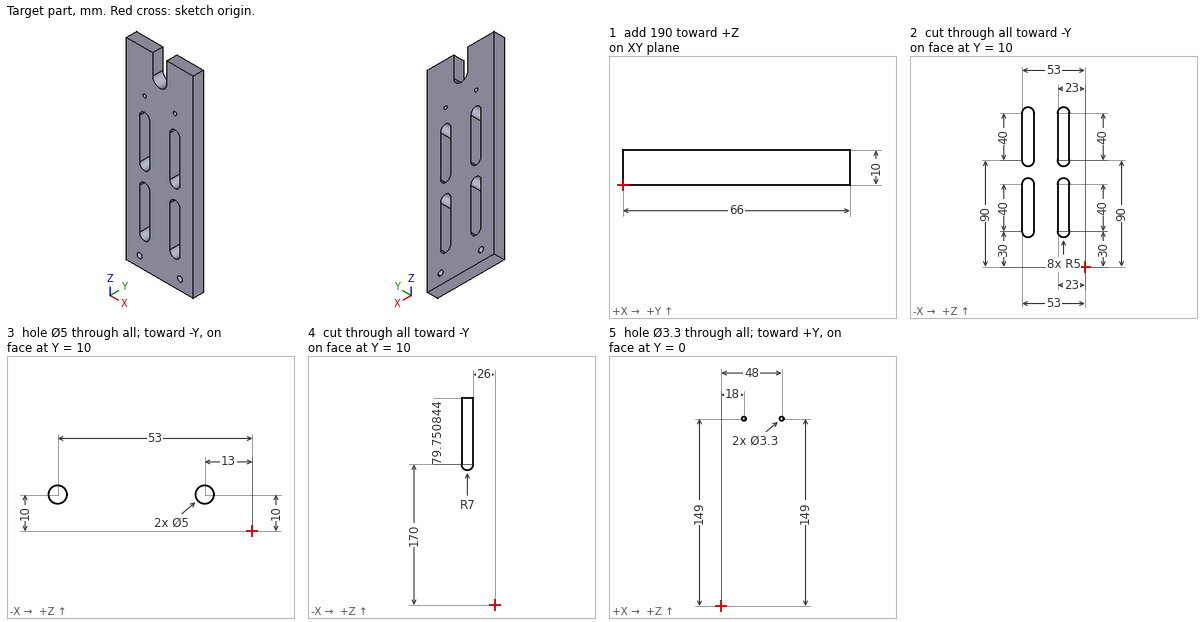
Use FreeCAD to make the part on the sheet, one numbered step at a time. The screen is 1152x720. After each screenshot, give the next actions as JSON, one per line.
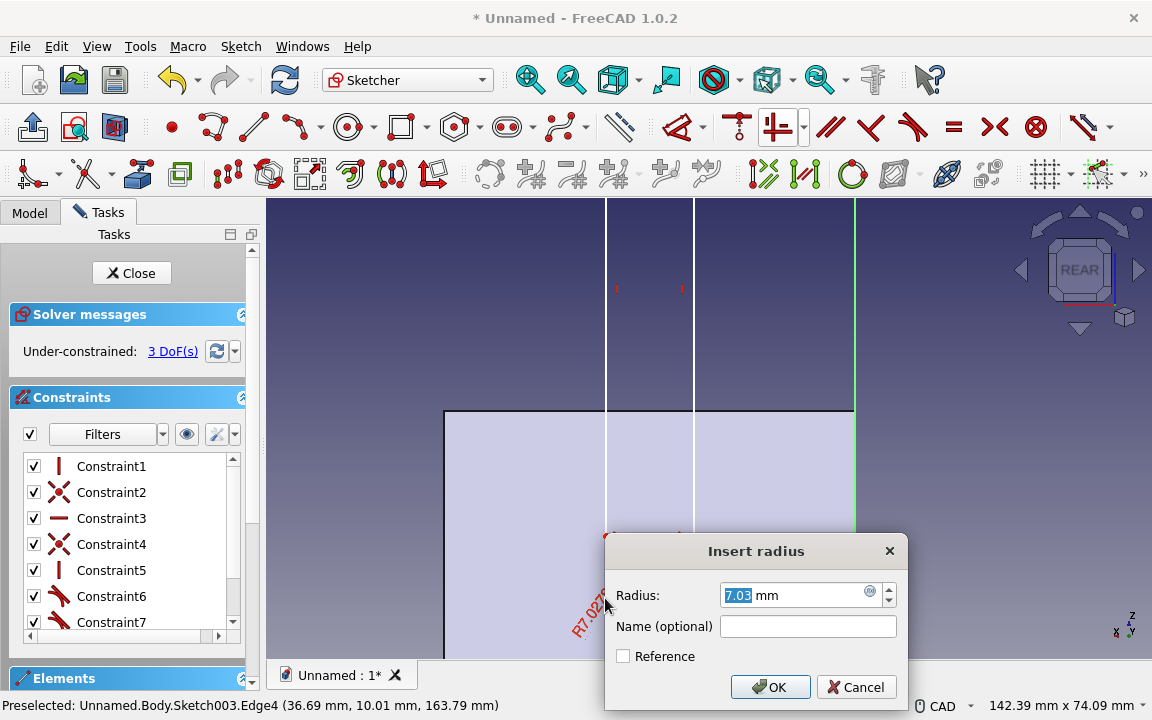
{"action": "type", "text": "7"}
{"action": "key", "text": "Return"}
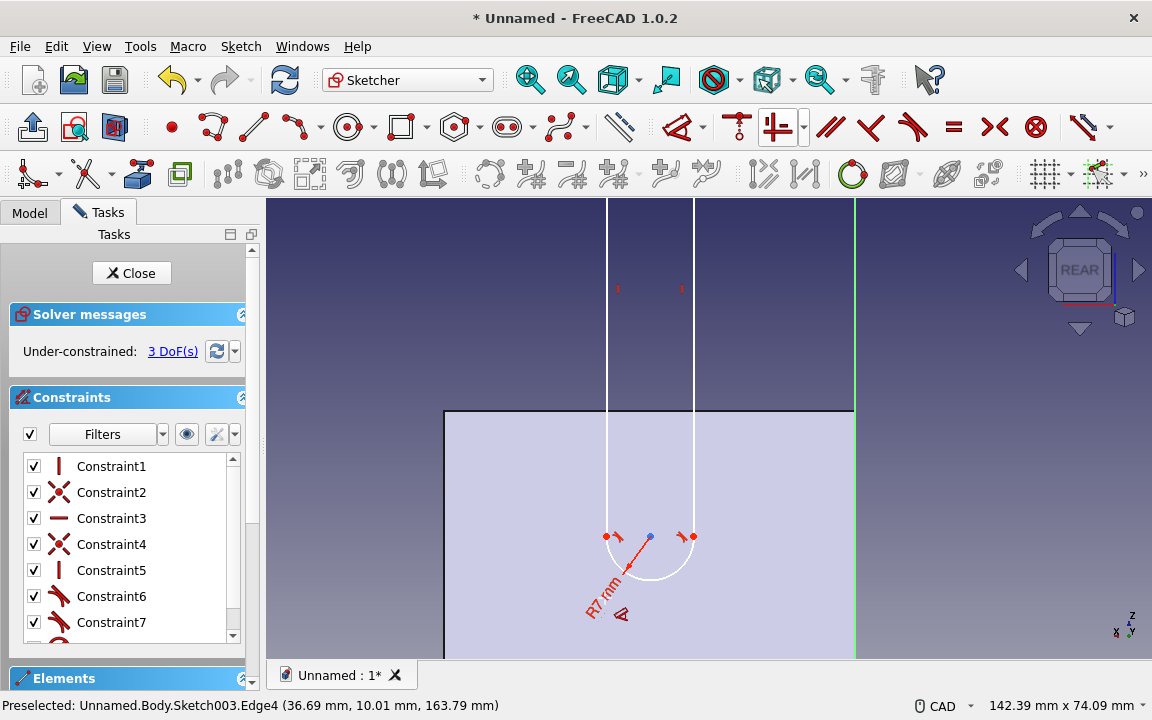
{"action": "left_click", "coordinate": [694, 537]}
{"action": "left_click", "coordinate": [774, 503]}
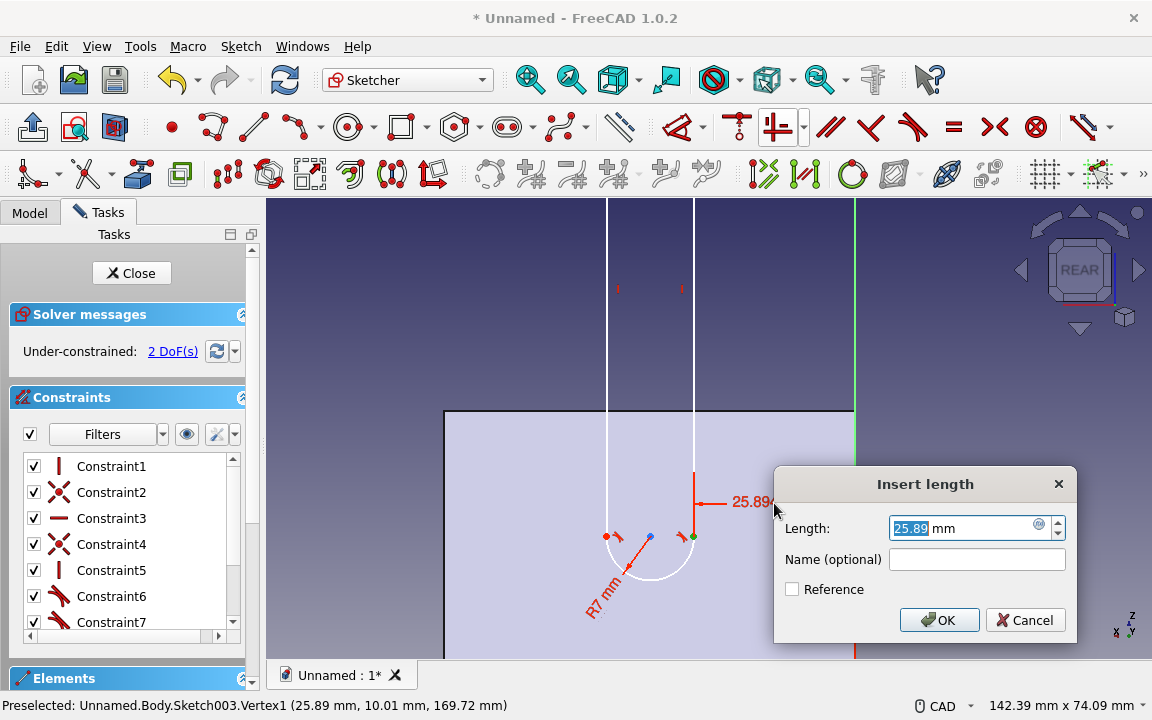
{"action": "type", "text": "26"}
{"action": "key", "text": "Return"}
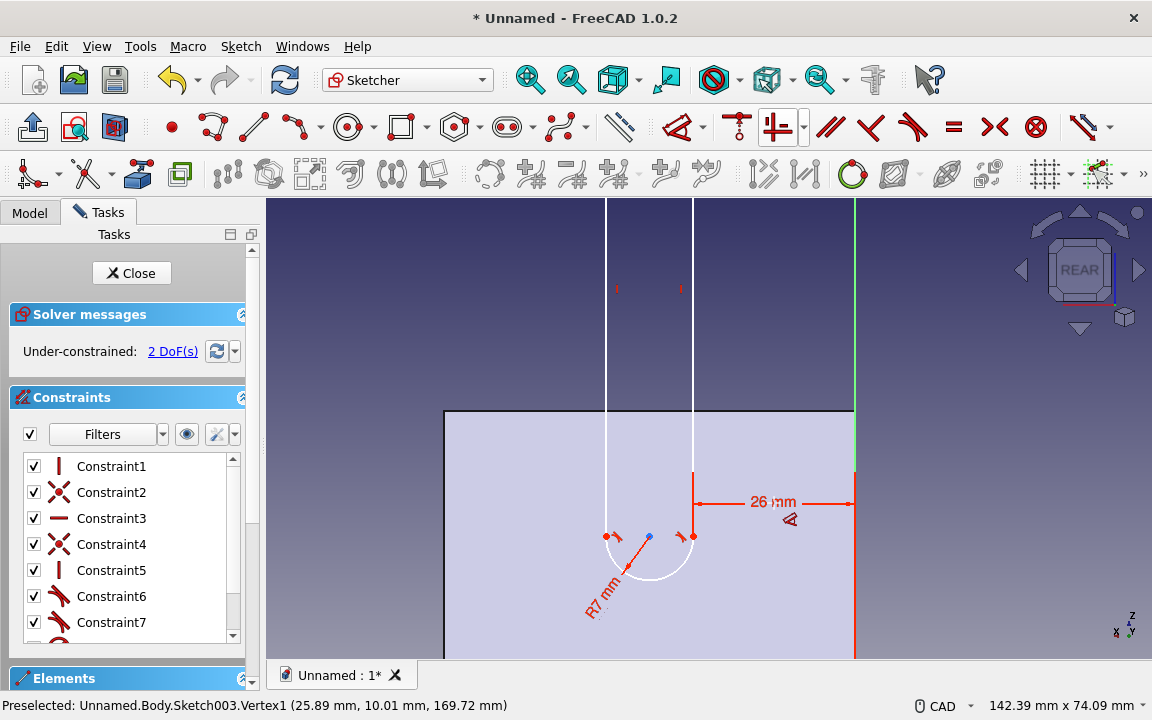
{"action": "left_click", "coordinate": [693, 537]}
{"action": "left_click", "coordinate": [889, 584]}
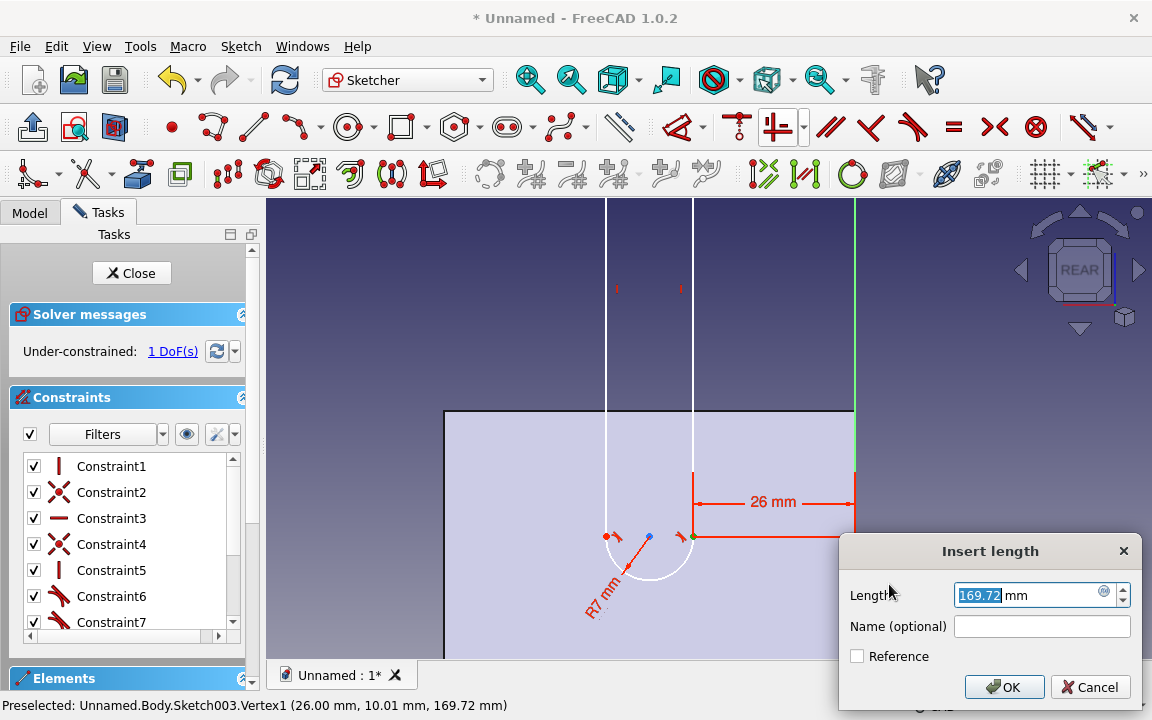
{"action": "type", "text": "170"}
{"action": "key", "text": "Return"}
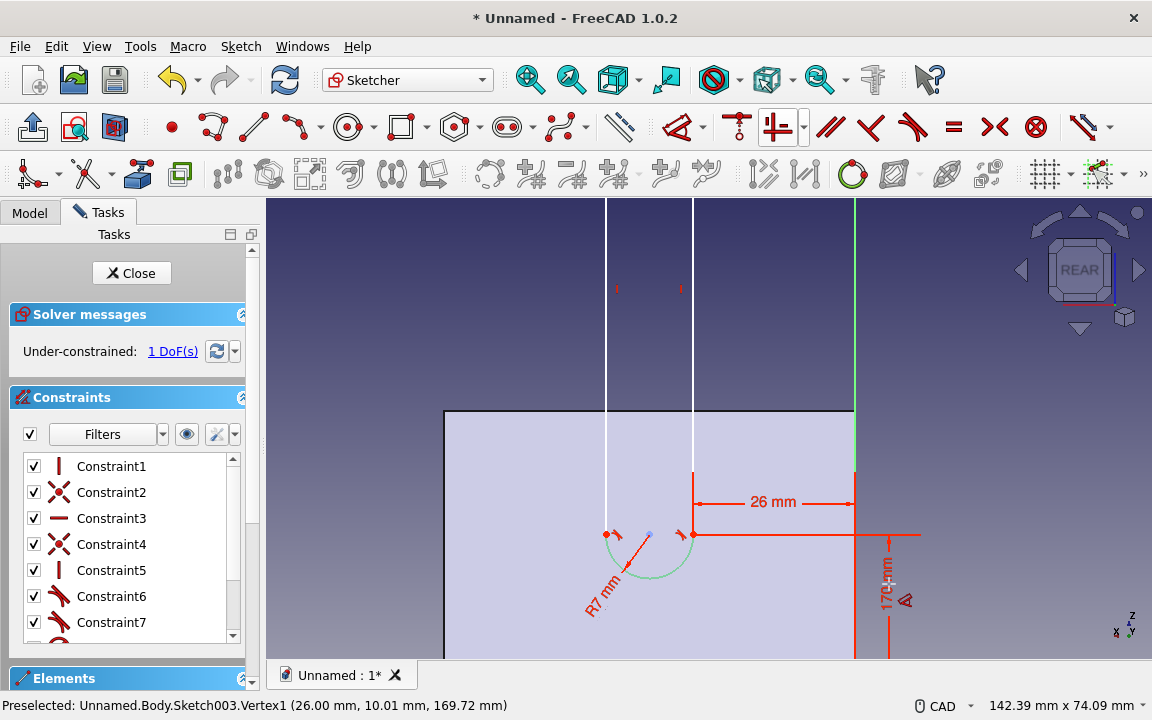
{"action": "left_click", "coordinate": [693, 387]}
{"action": "left_click", "coordinate": [727, 380]}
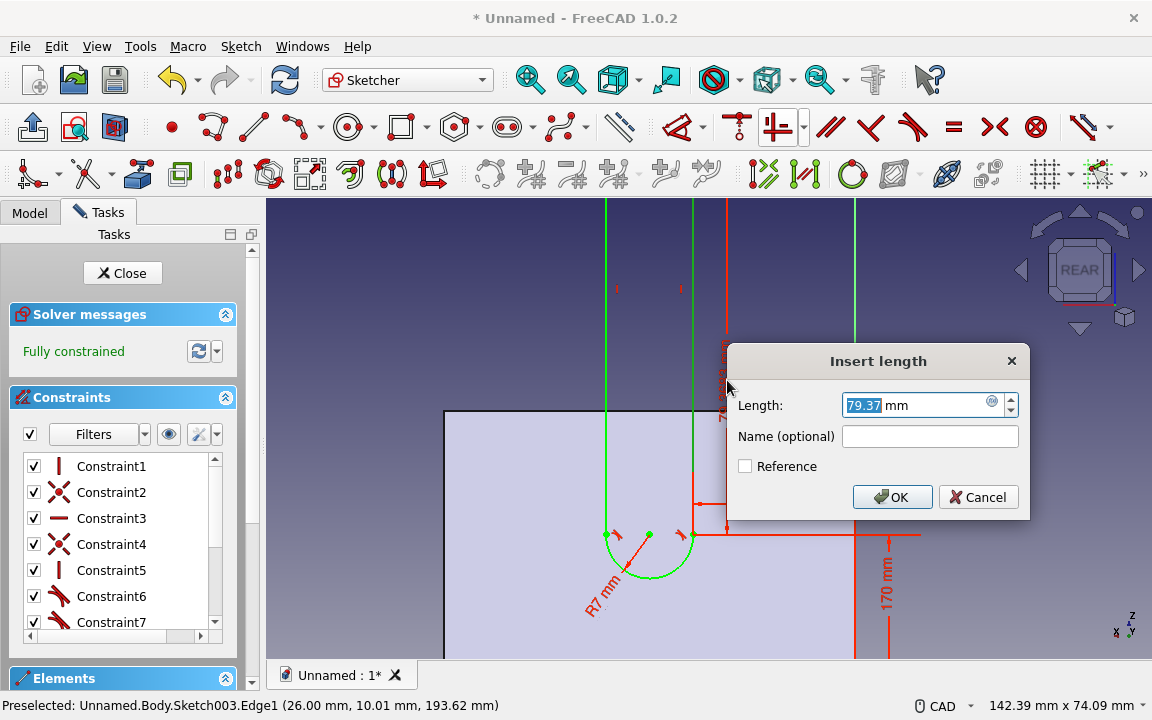
{"action": "type", "text": "79.750844"}
{"action": "key", "text": "Return"}
{"action": "key", "text": "Escape"}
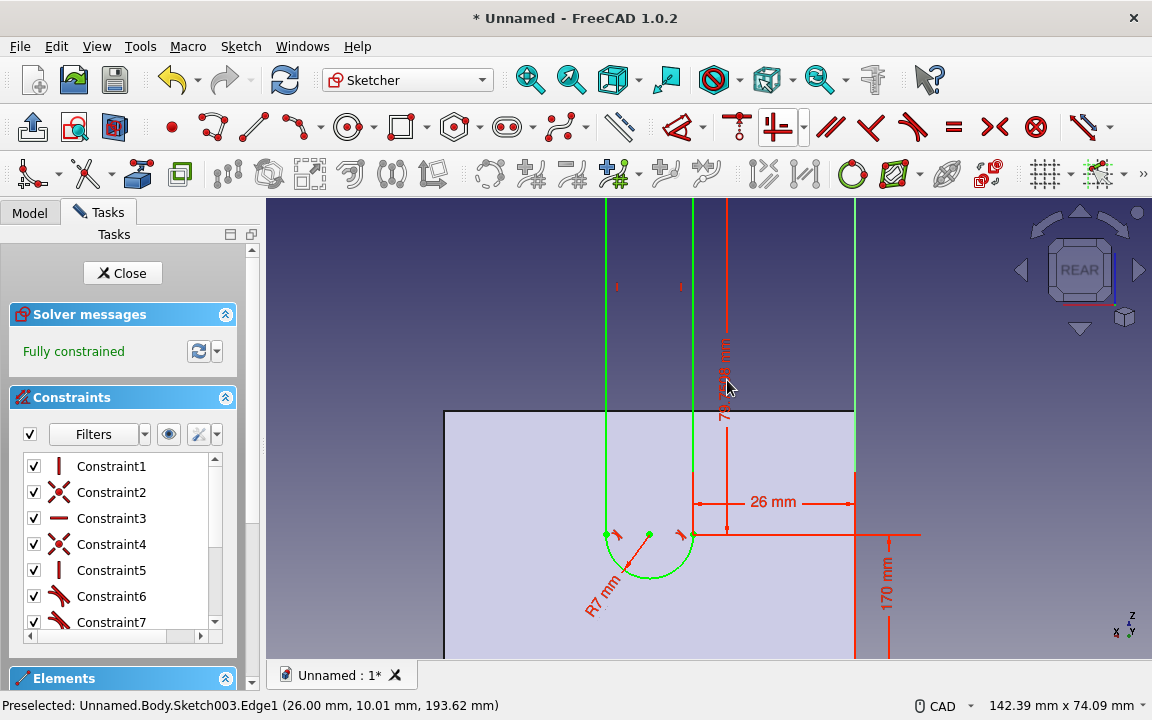
{"action": "left_click", "coordinate": [123, 273]}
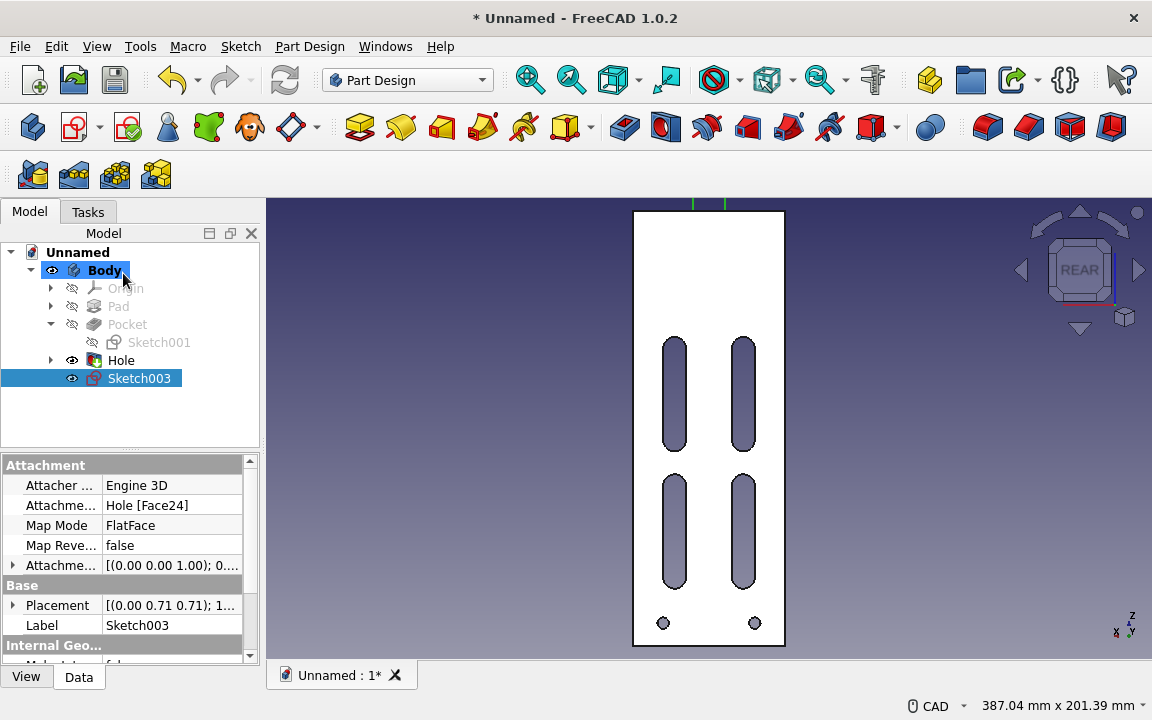
{"action": "left_click", "coordinate": [625, 128]}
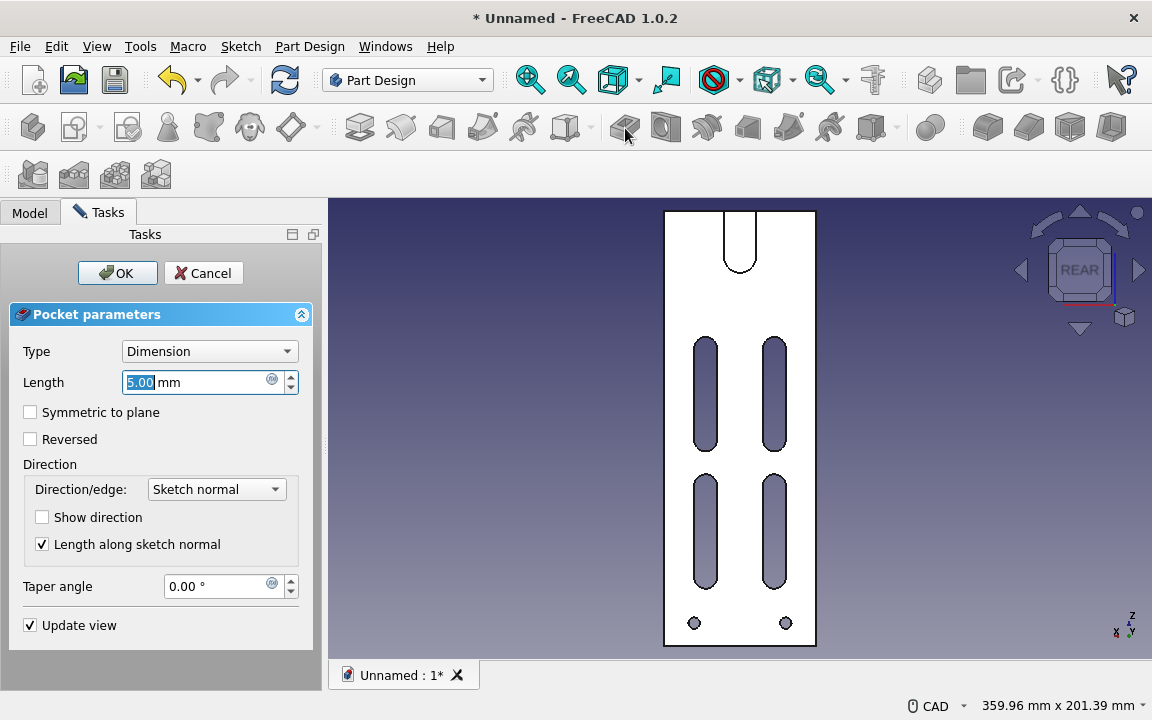
{"action": "left_click", "coordinate": [210, 352]}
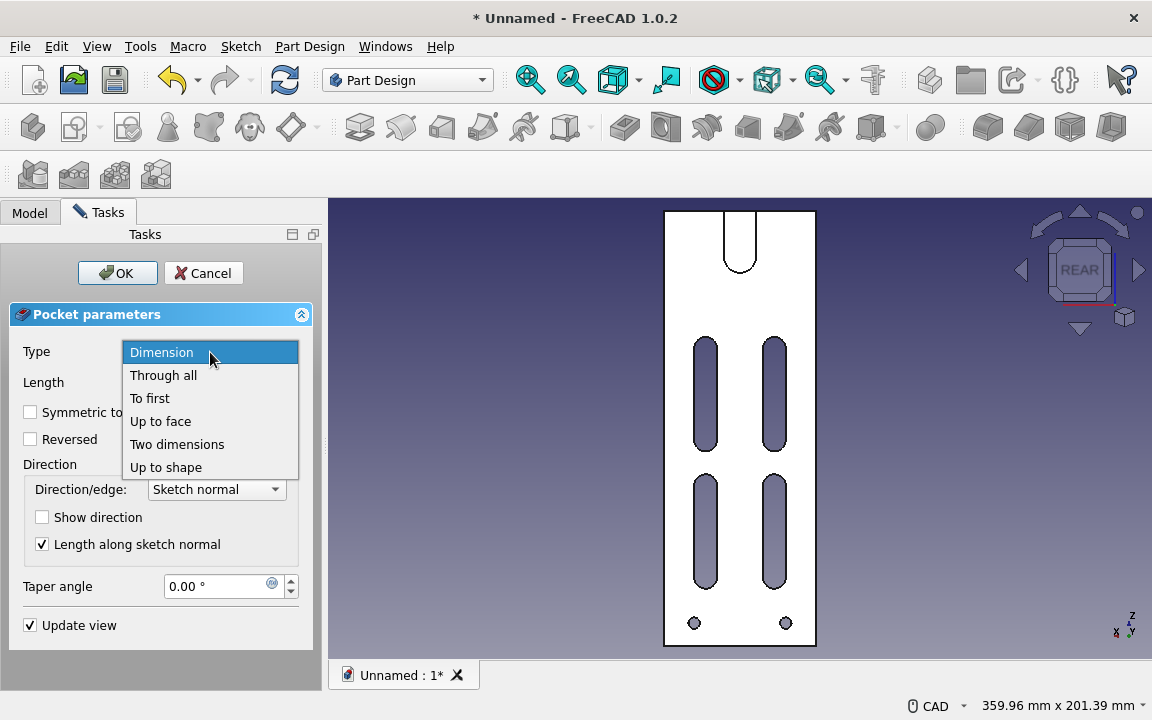
{"action": "left_click", "coordinate": [208, 376]}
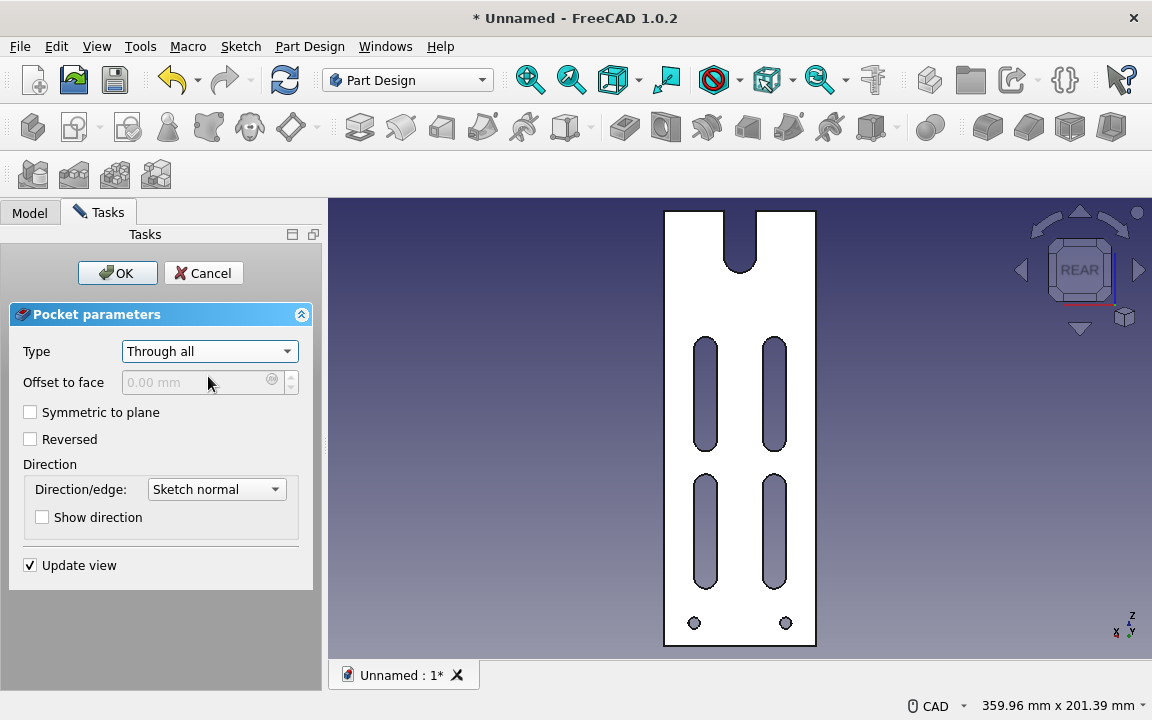
{"action": "left_click", "coordinate": [118, 273]}